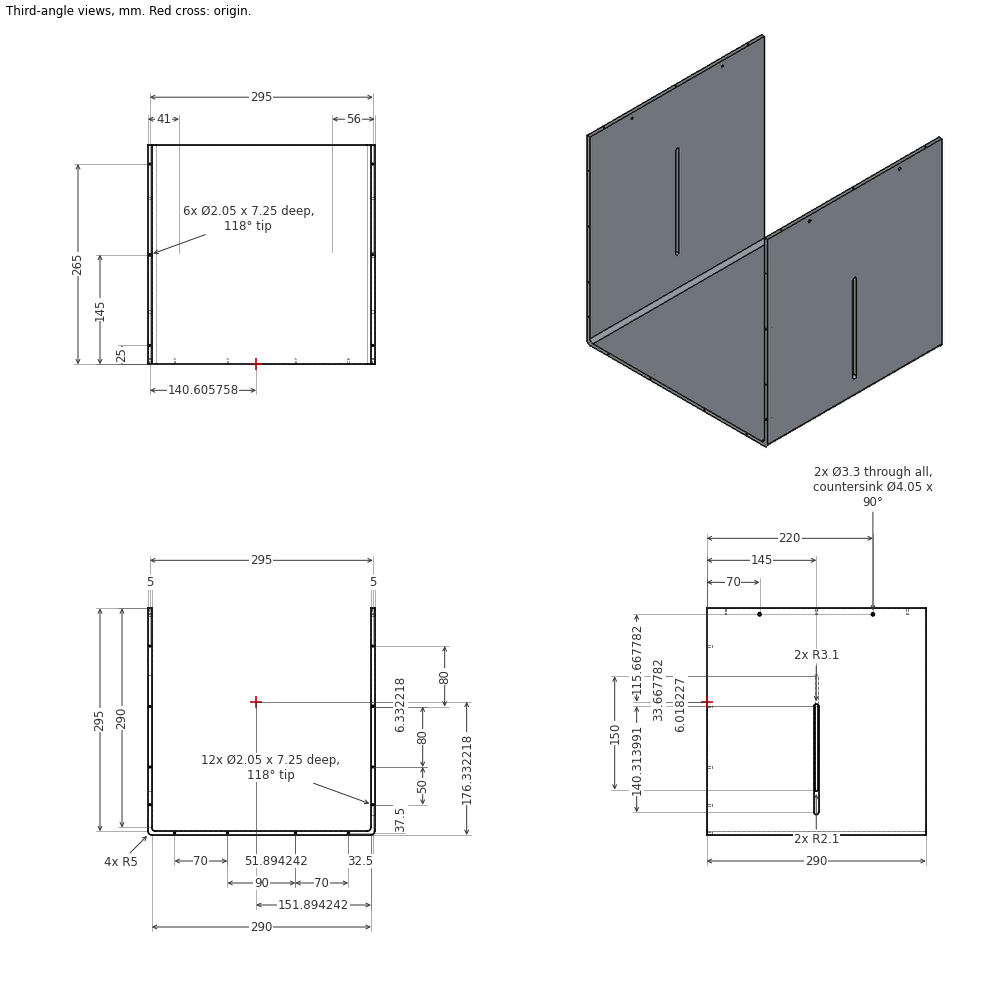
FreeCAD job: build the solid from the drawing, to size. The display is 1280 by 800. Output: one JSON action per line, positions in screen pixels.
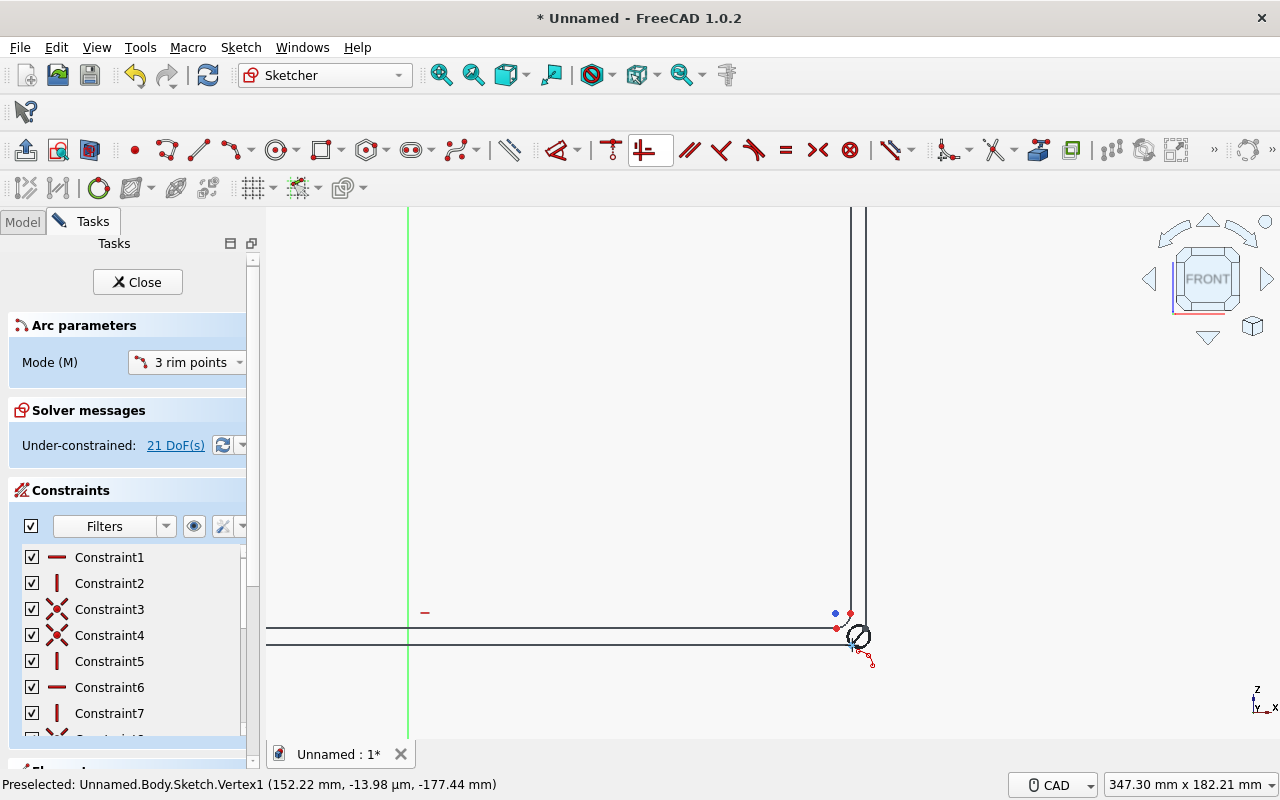
{"action": "scroll", "coordinate": [861, 638], "scroll_direction": "up", "scroll_amount": 7}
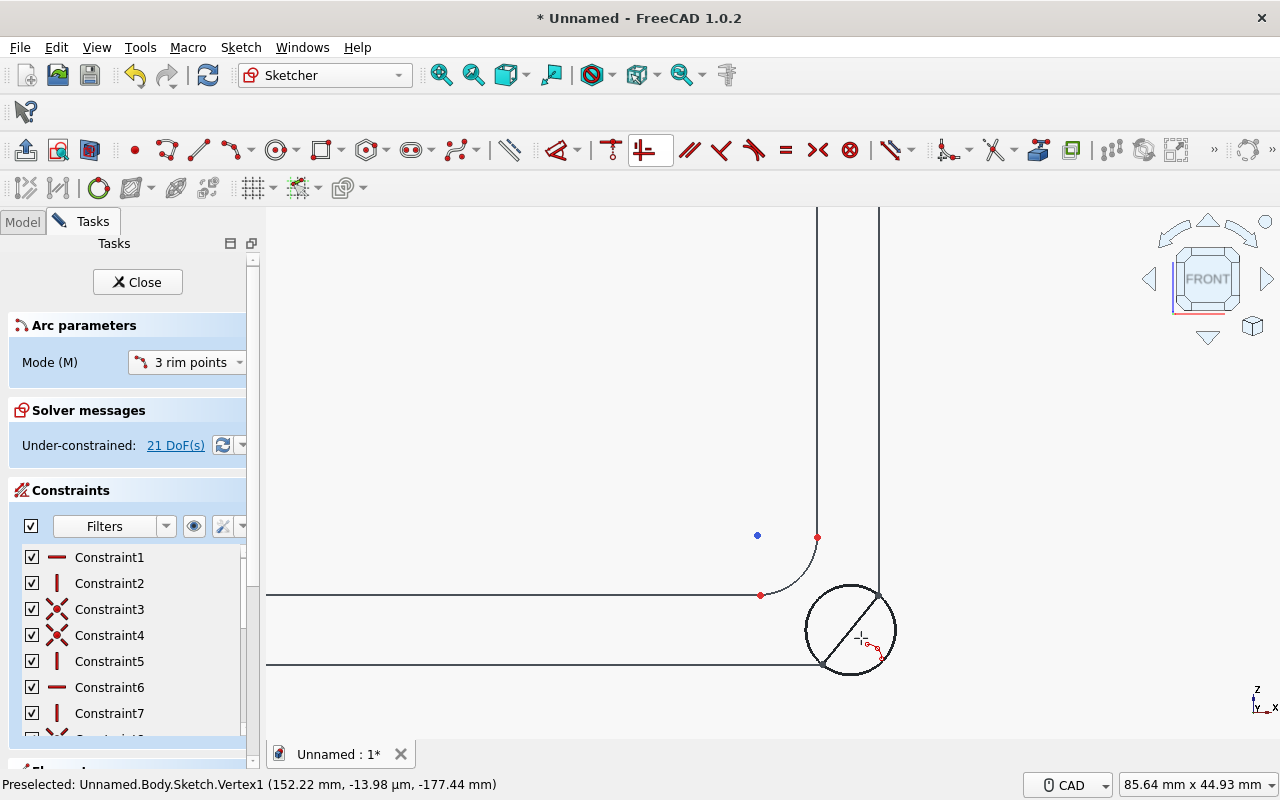
{"action": "left_click", "coordinate": [860, 634]}
{"action": "key", "text": "Escape"}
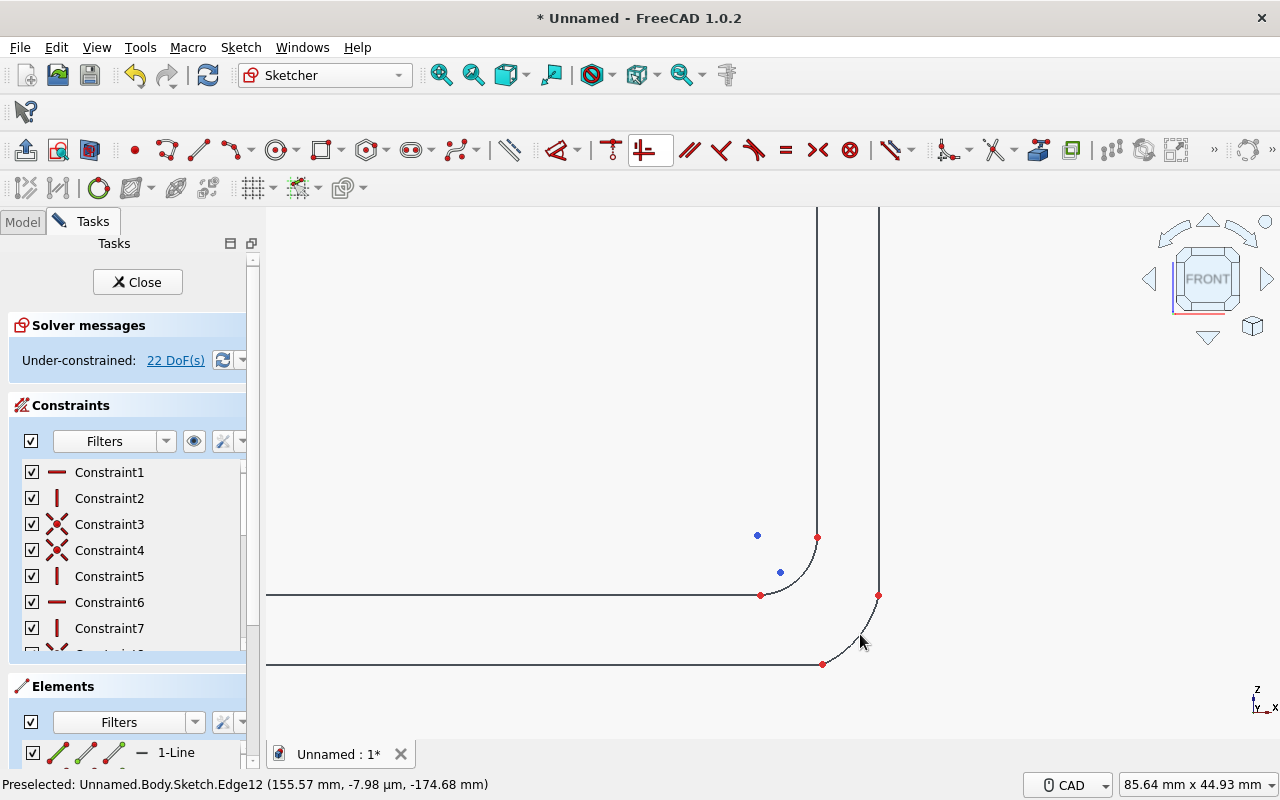
{"action": "scroll", "coordinate": [864, 632], "scroll_direction": "down", "scroll_amount": 12}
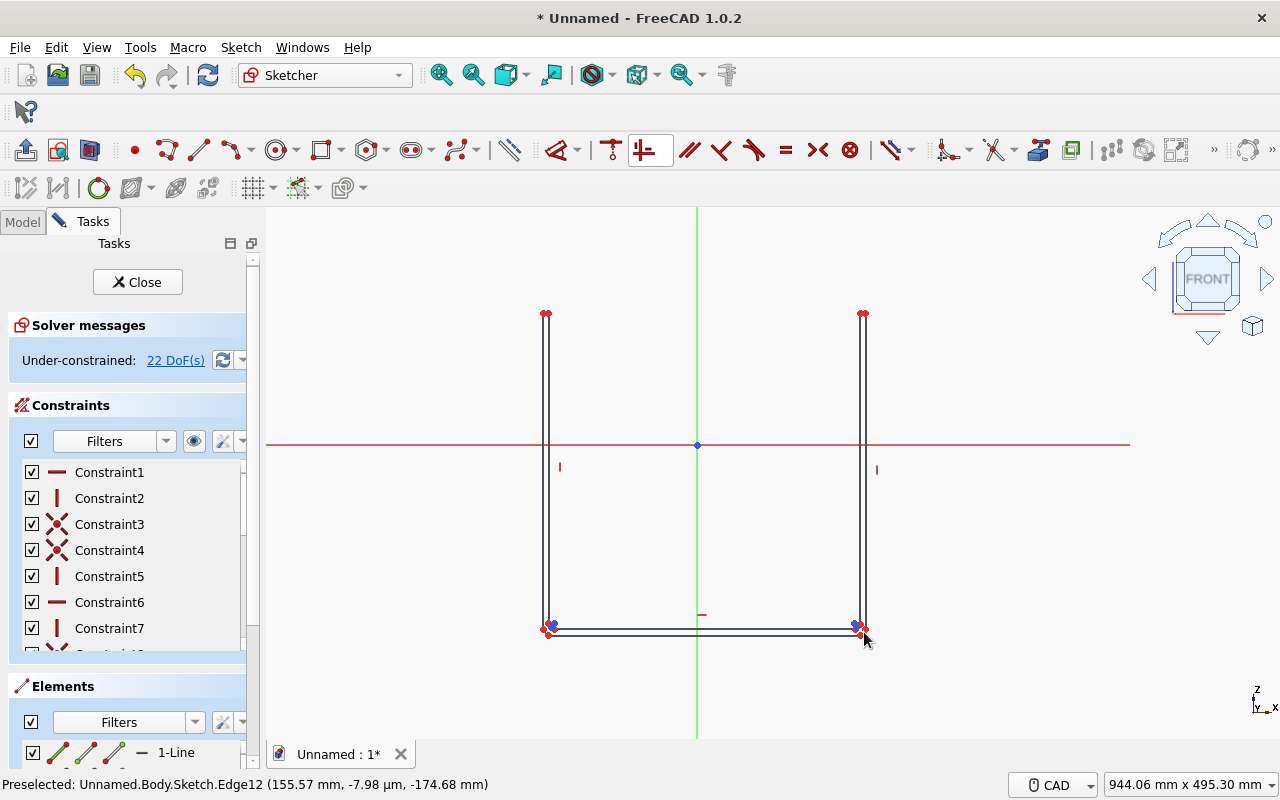
{"action": "scroll", "coordinate": [767, 636], "scroll_direction": "up", "scroll_amount": 4}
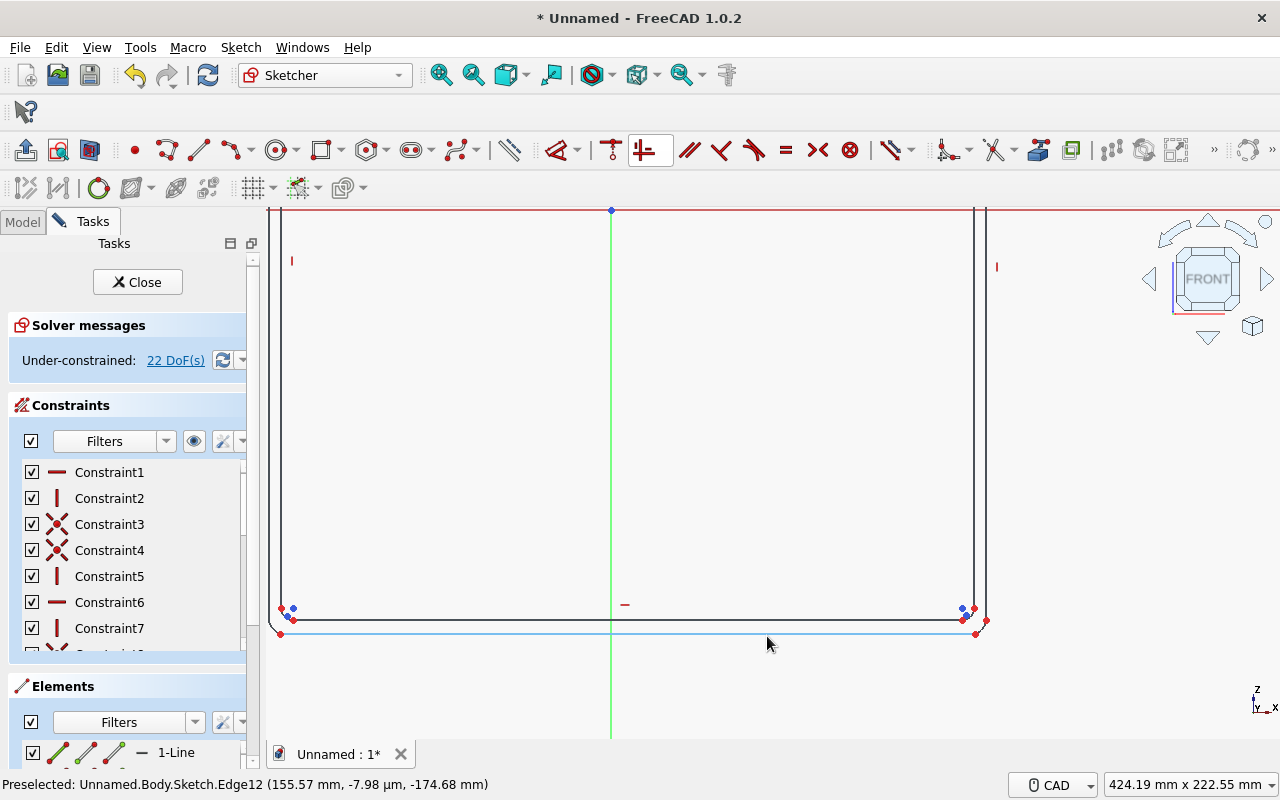
{"action": "left_click", "coordinate": [767, 634]}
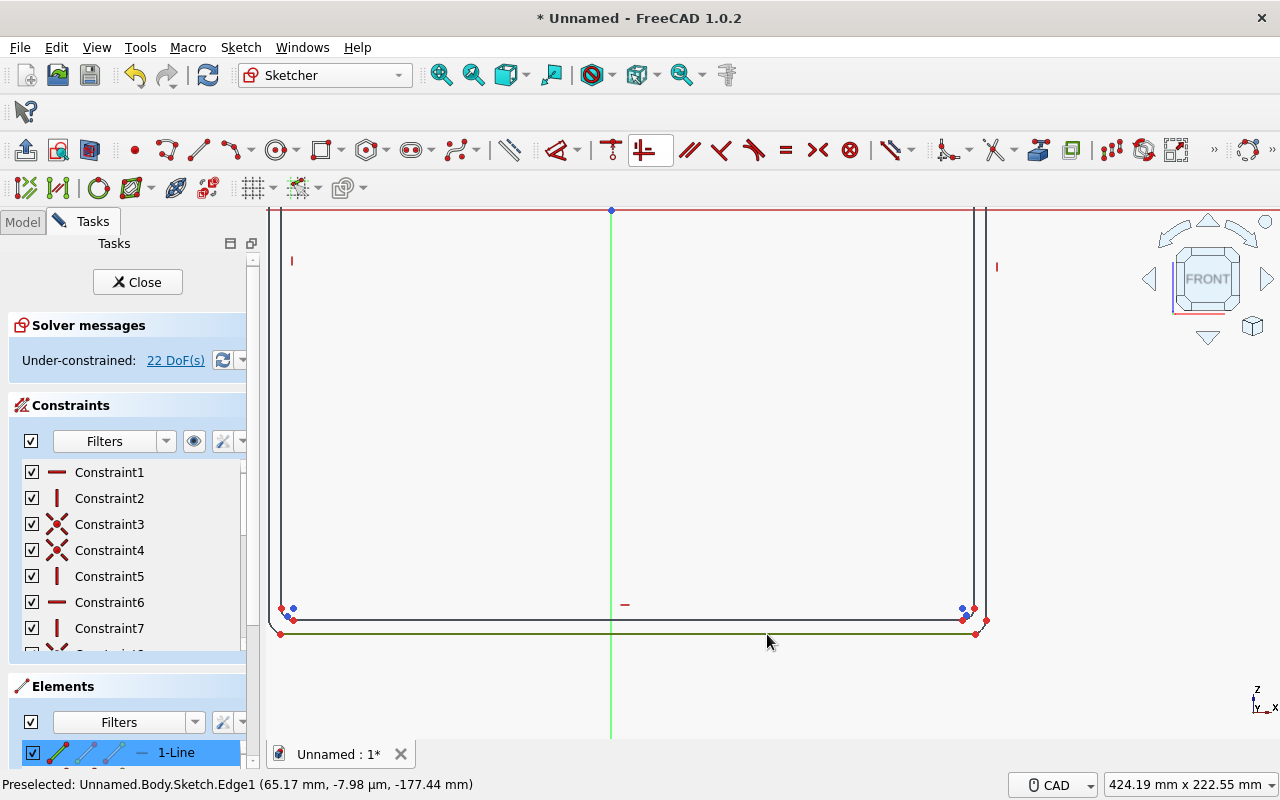
{"action": "scroll", "coordinate": [767, 636], "scroll_direction": "down", "scroll_amount": 4}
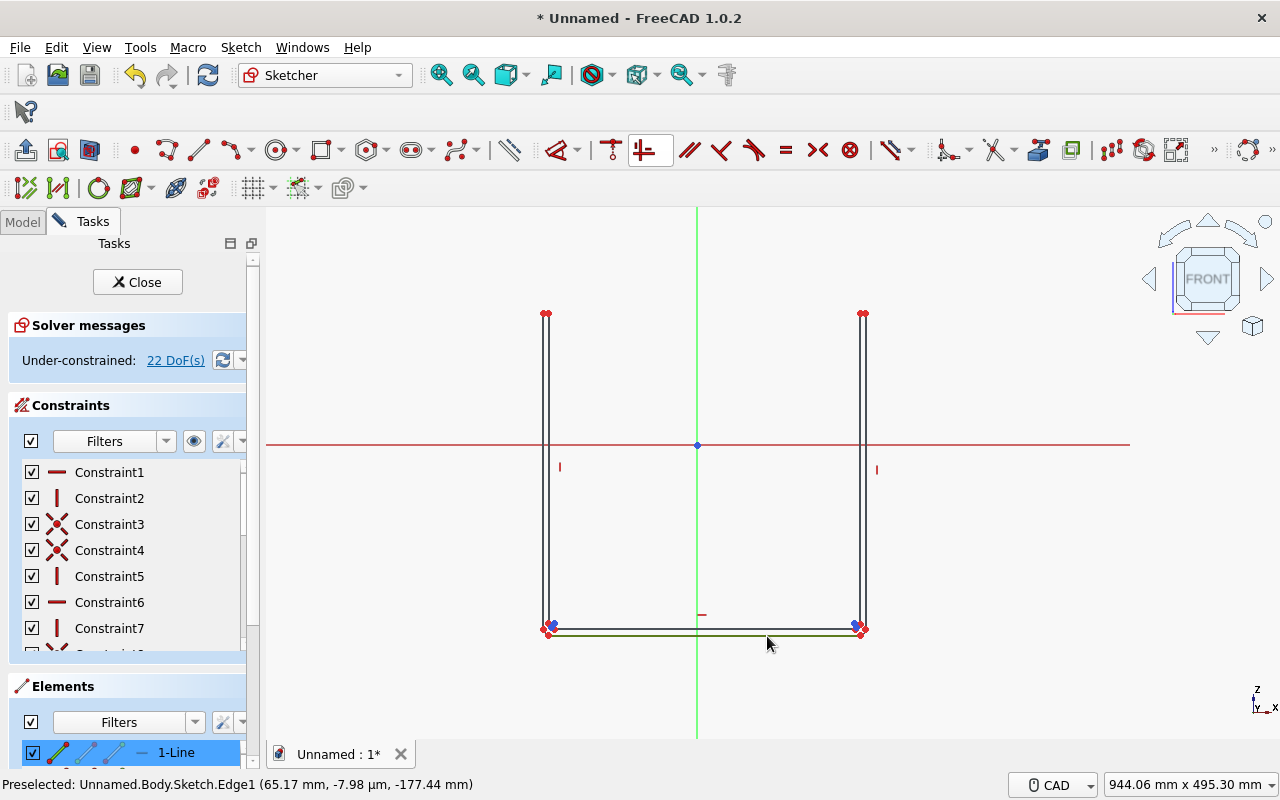
{"action": "scroll", "coordinate": [545, 633], "scroll_direction": "up", "scroll_amount": 6}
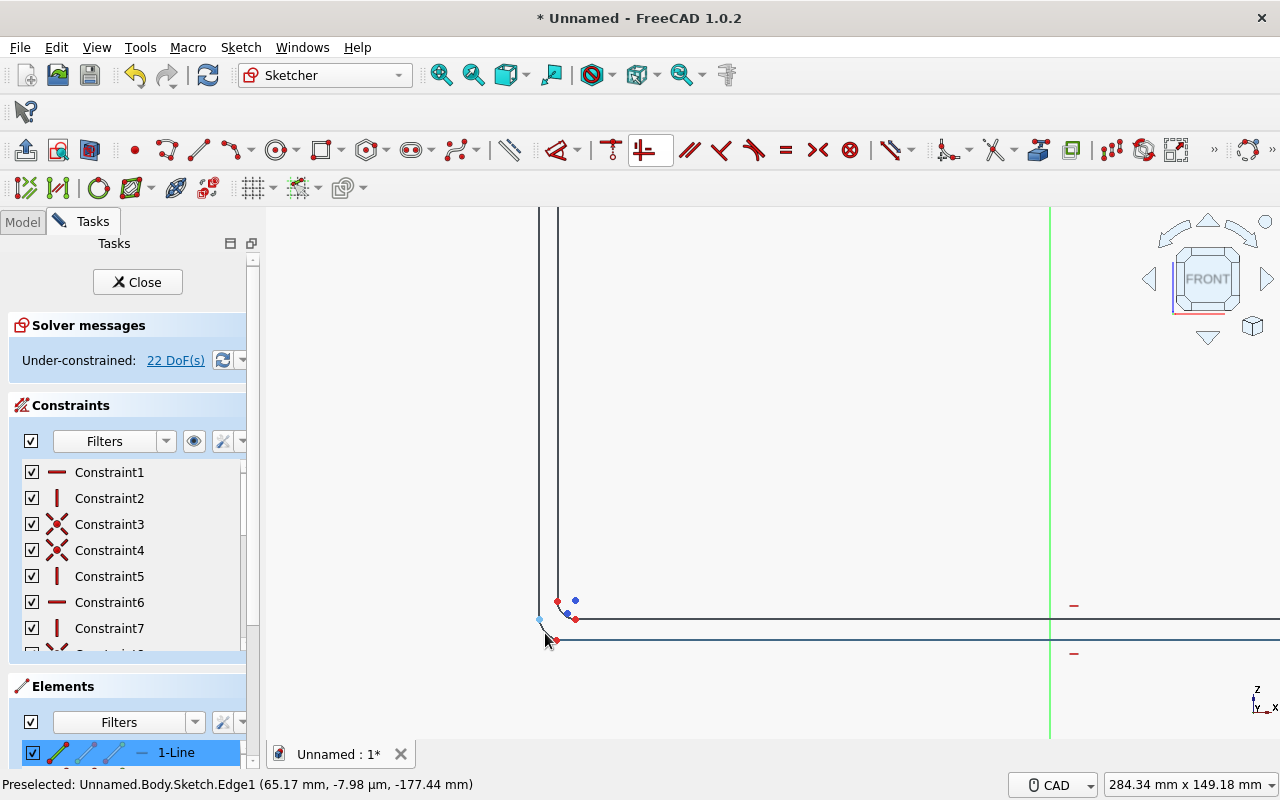
{"action": "left_click", "coordinate": [546, 632]}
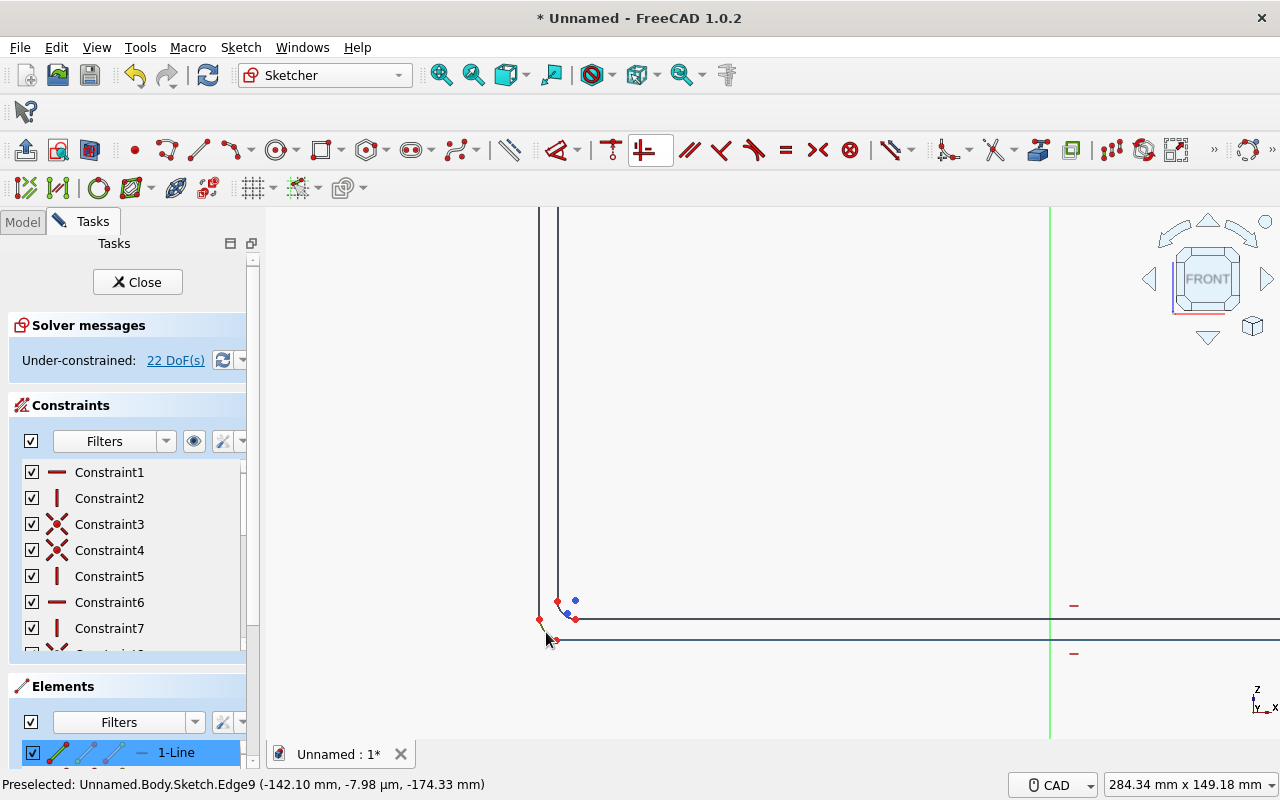
{"action": "left_click", "coordinate": [754, 150]}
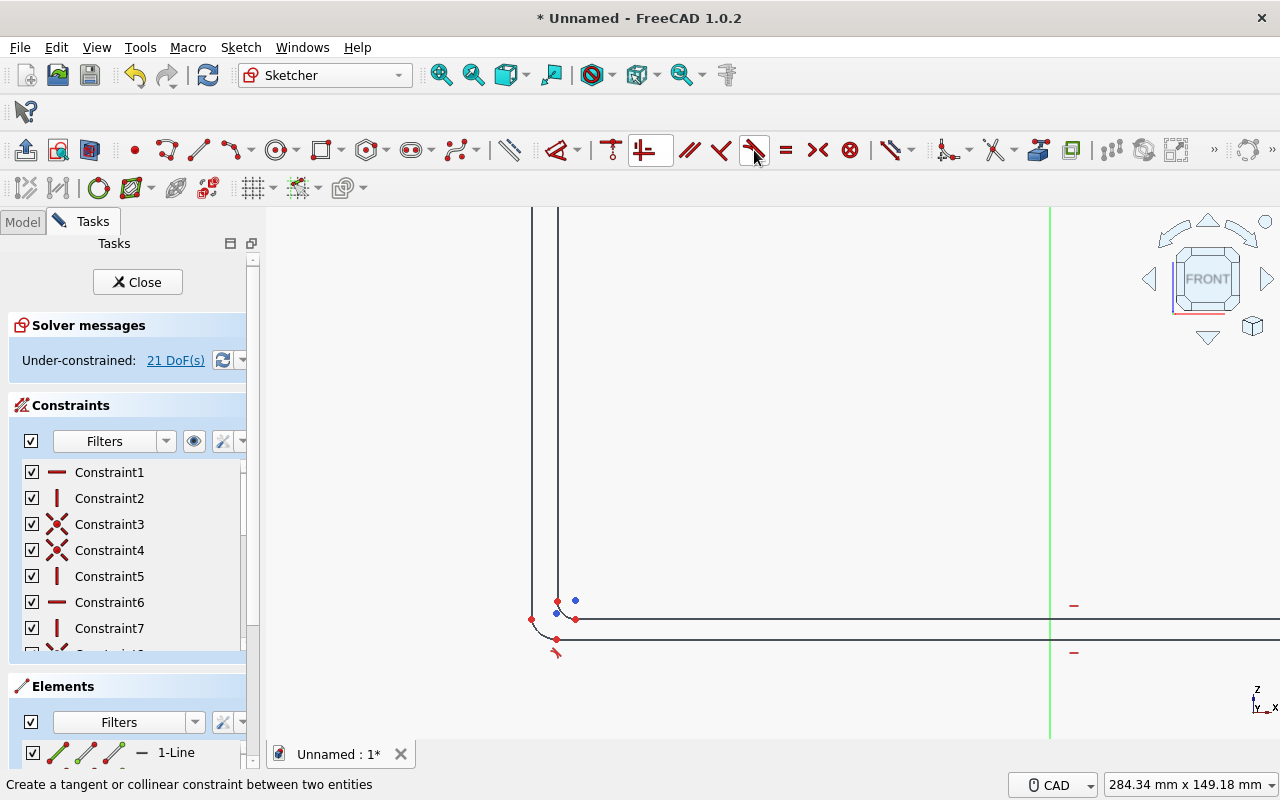
{"action": "left_click", "coordinate": [868, 640]}